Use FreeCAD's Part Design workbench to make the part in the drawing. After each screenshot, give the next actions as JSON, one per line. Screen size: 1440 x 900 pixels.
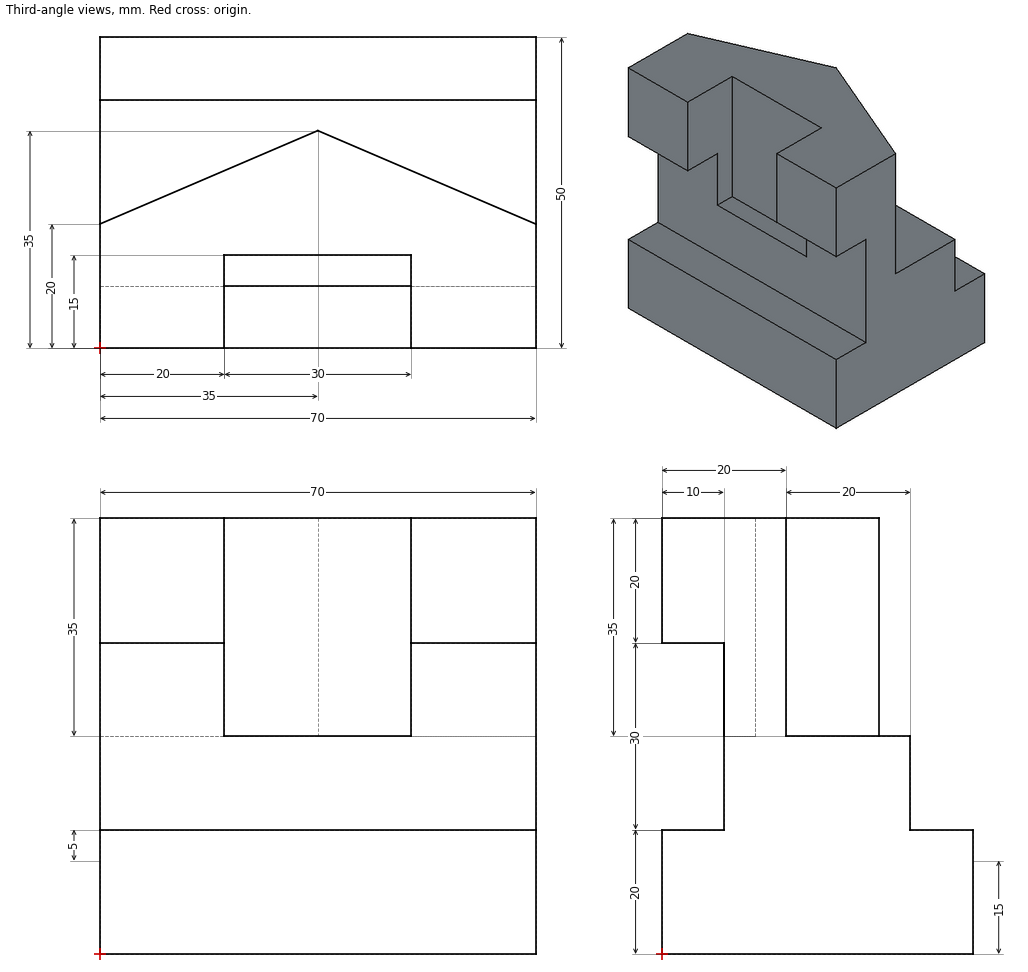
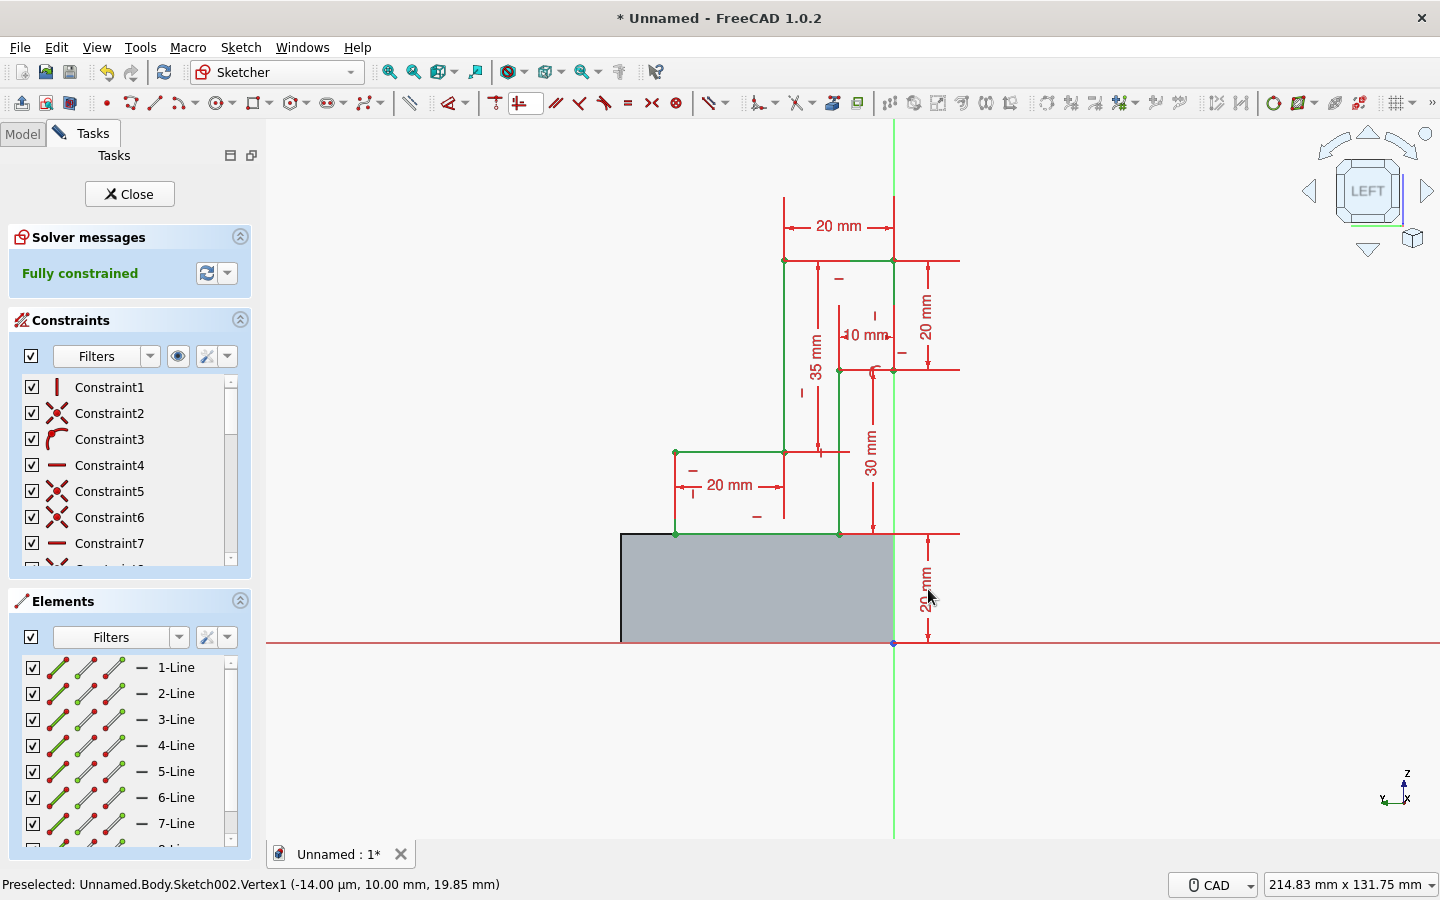
{"action": "left_click", "coordinate": [130, 194]}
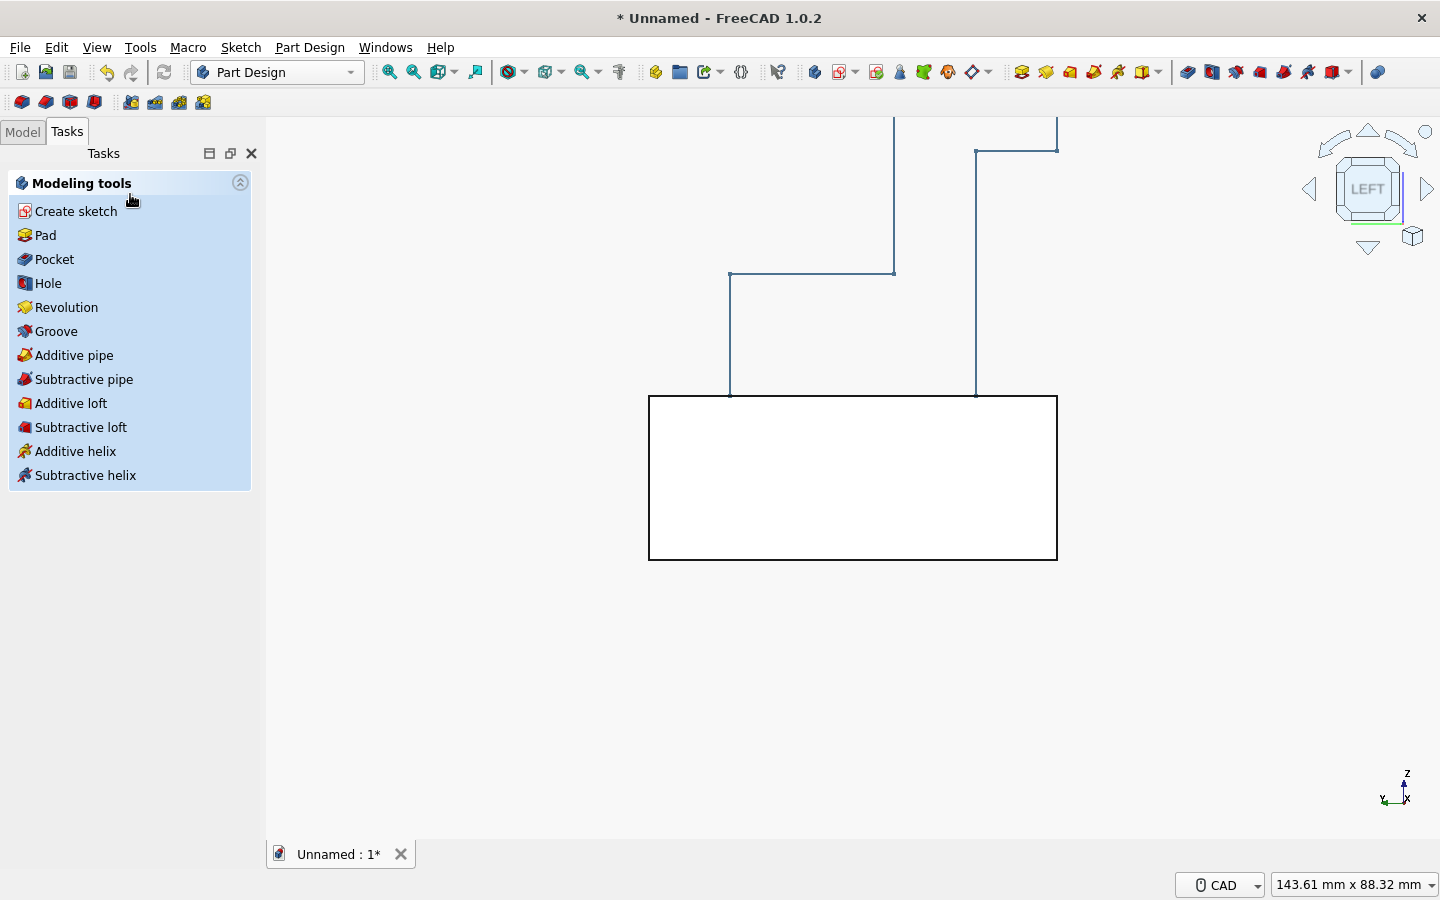
{"action": "left_click", "coordinate": [1022, 72]}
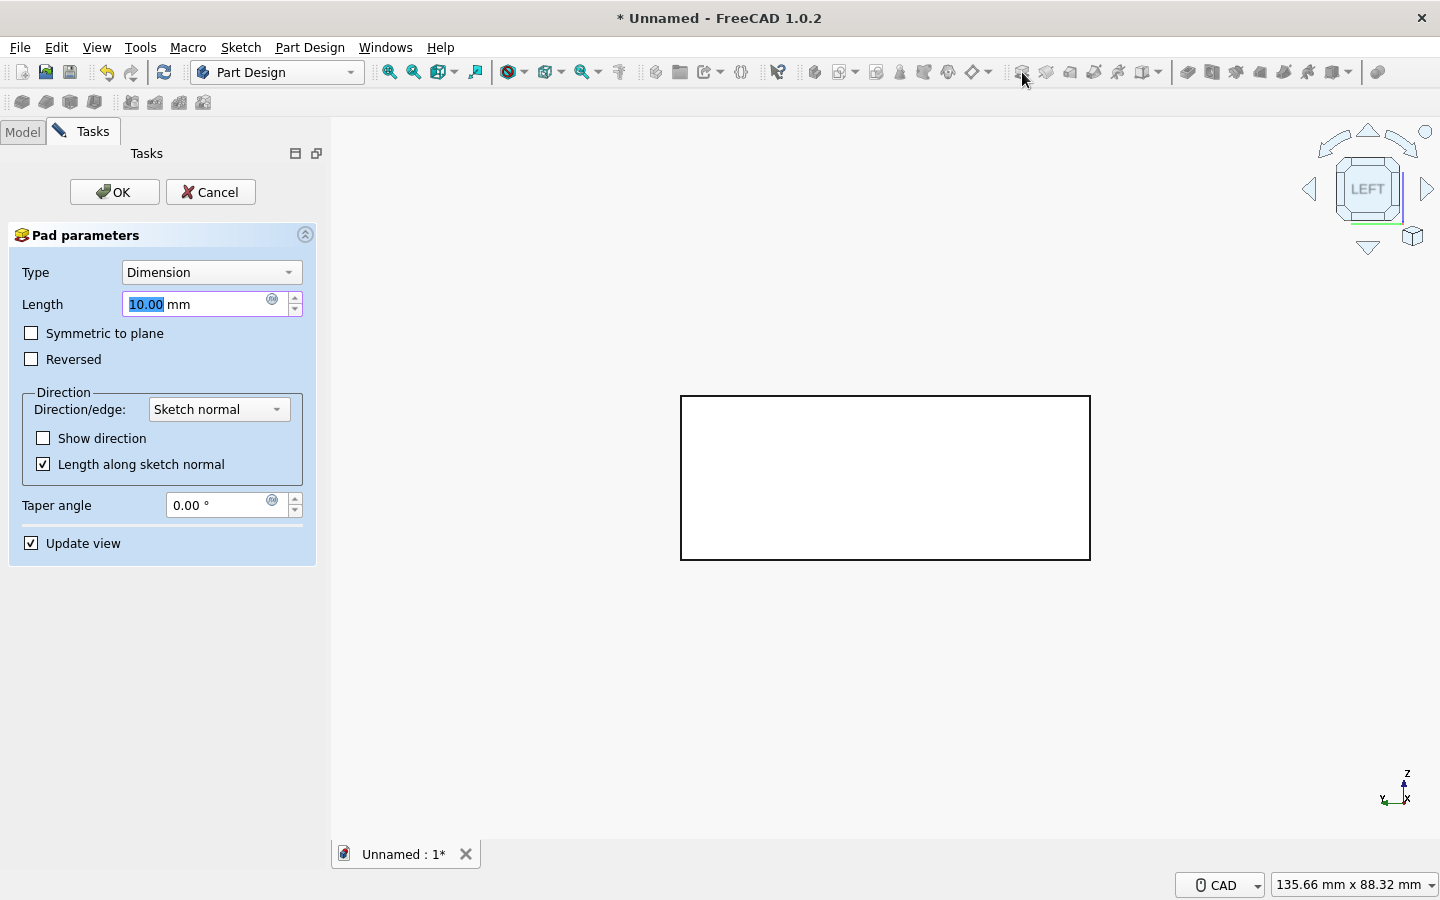
{"action": "type", "text": "70"}
{"action": "key", "text": "Tab"}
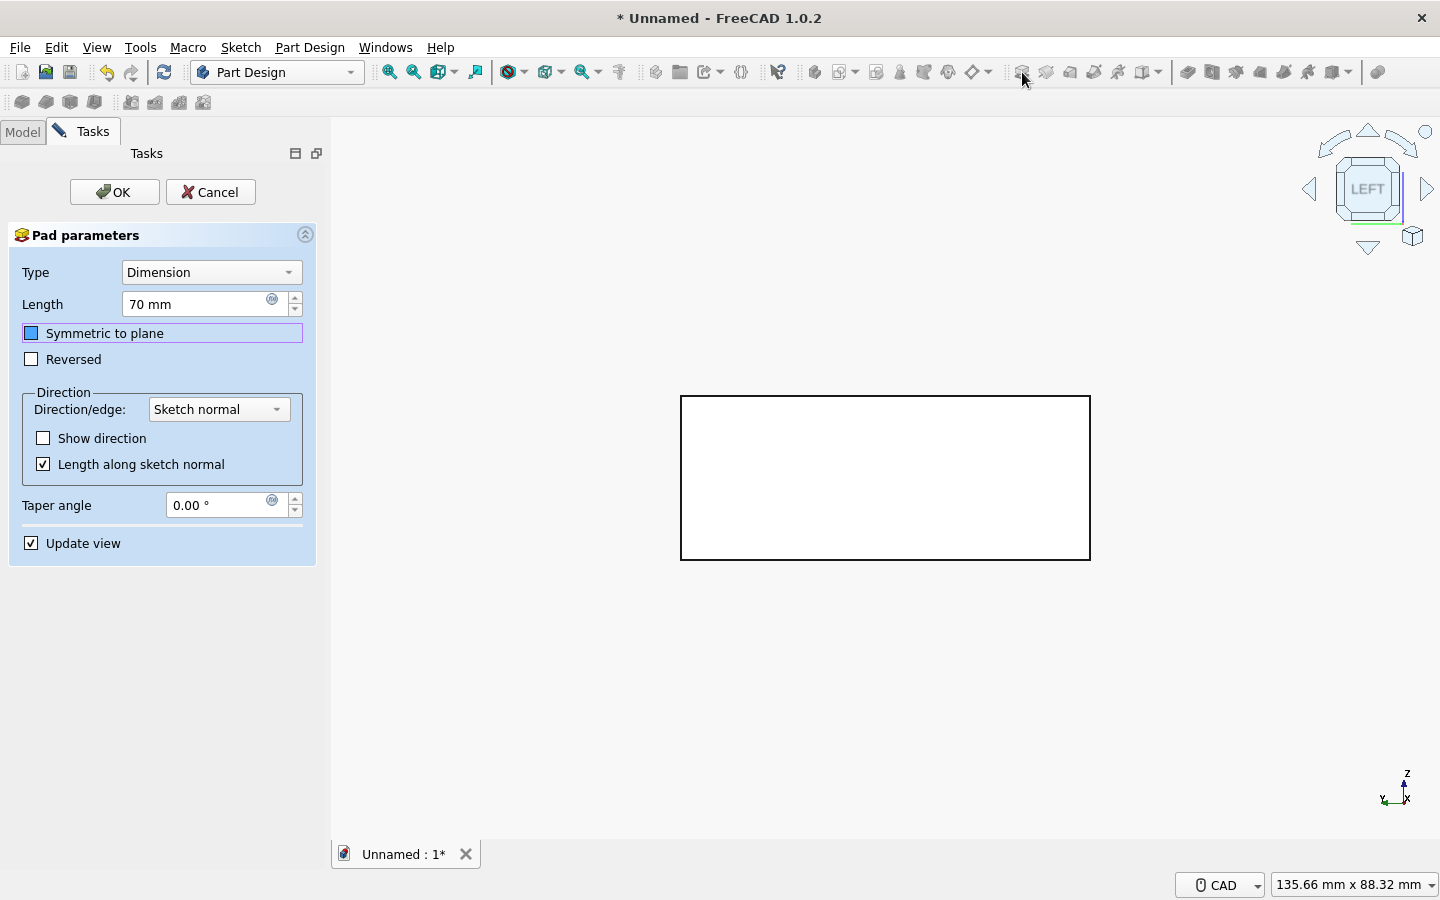
{"action": "left_click", "coordinate": [30, 359]}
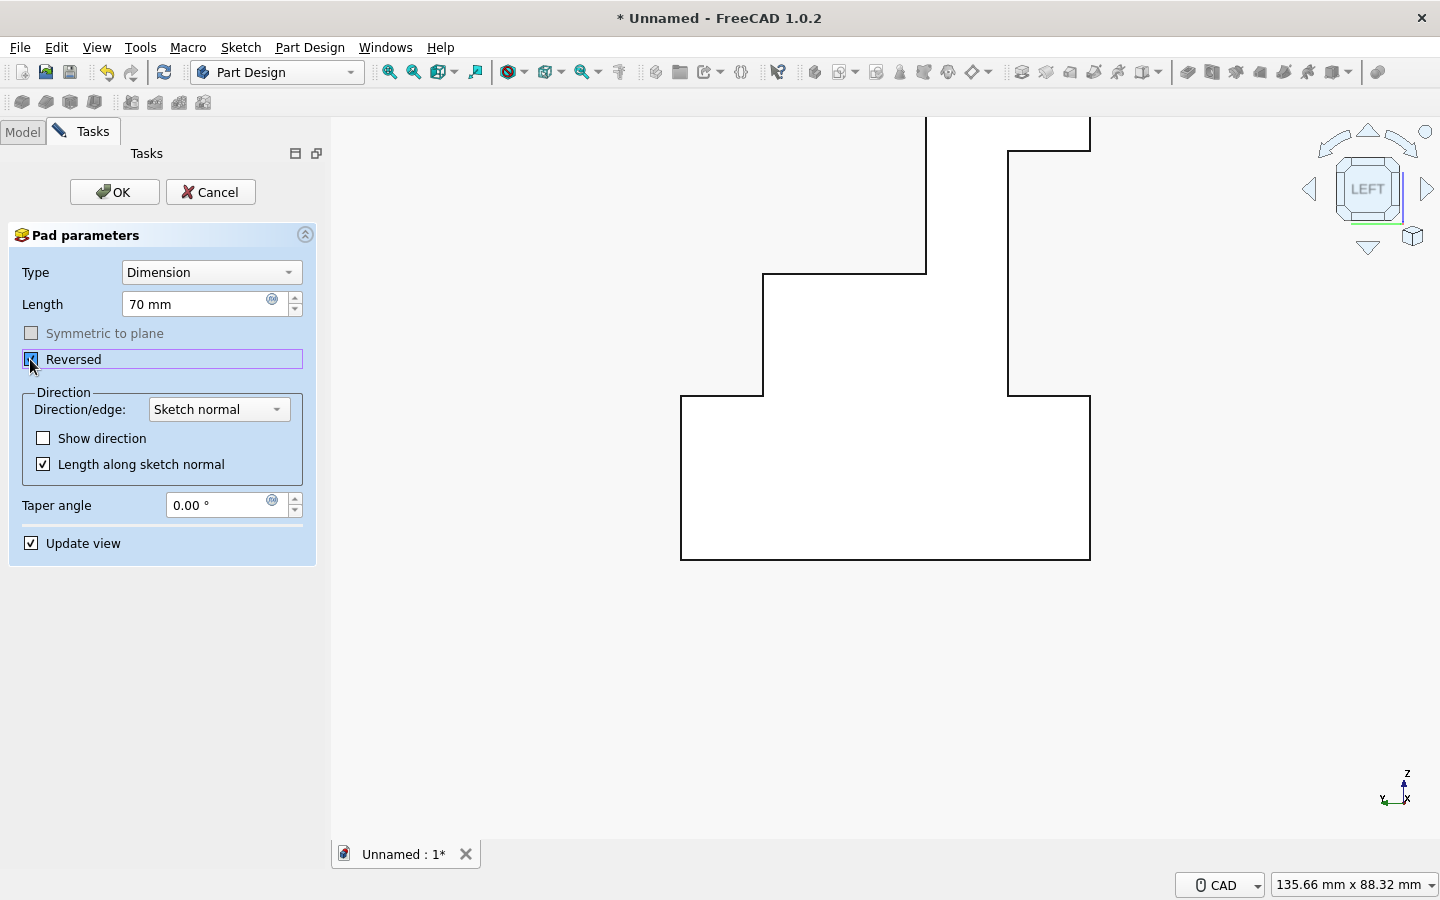
{"action": "left_click", "coordinate": [115, 192]}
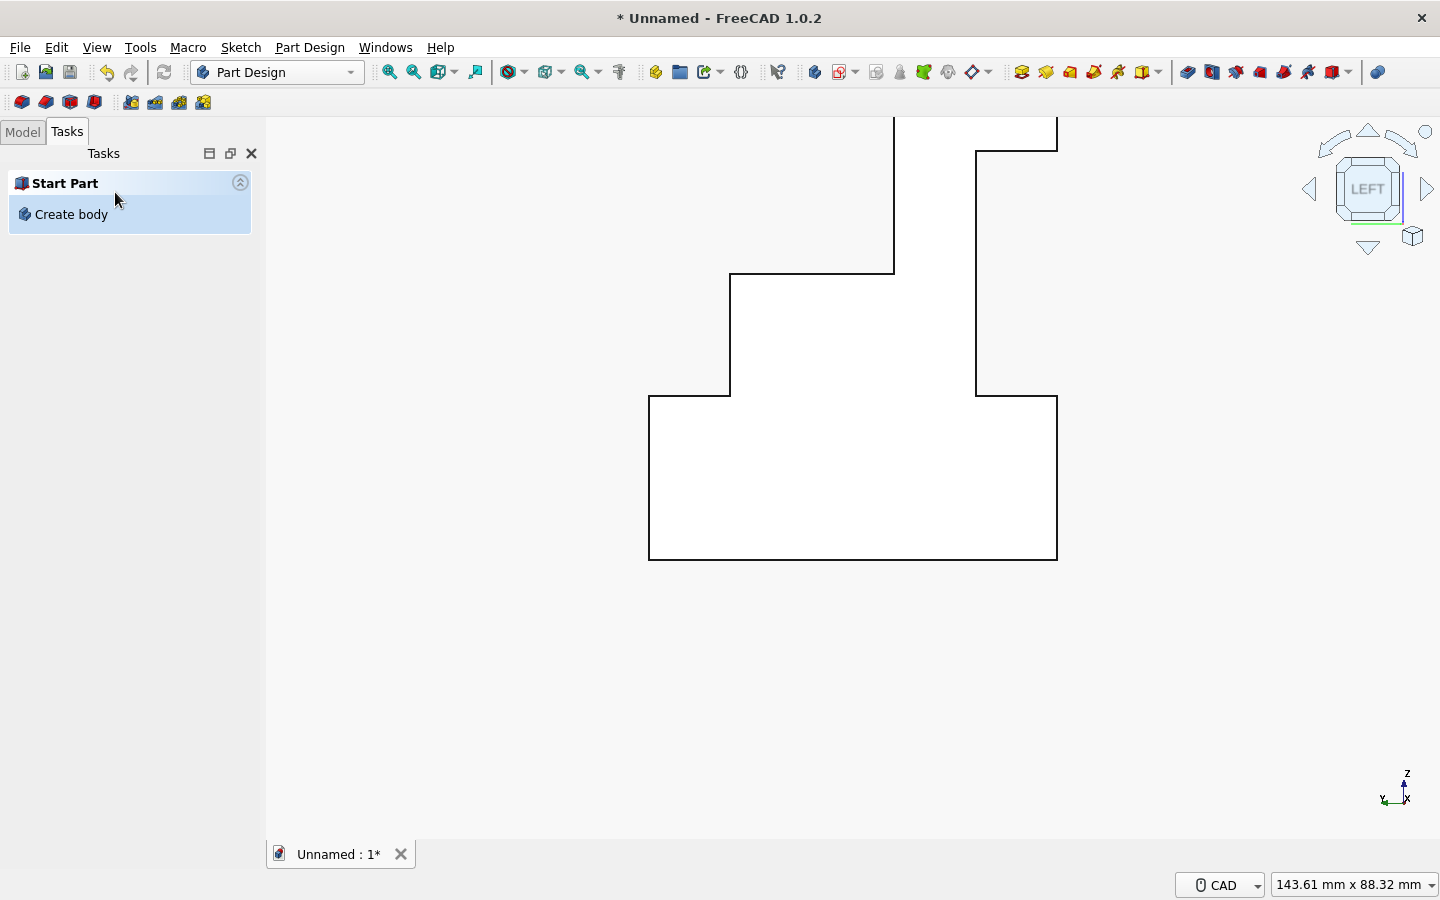
{"action": "left_click", "coordinate": [390, 72]}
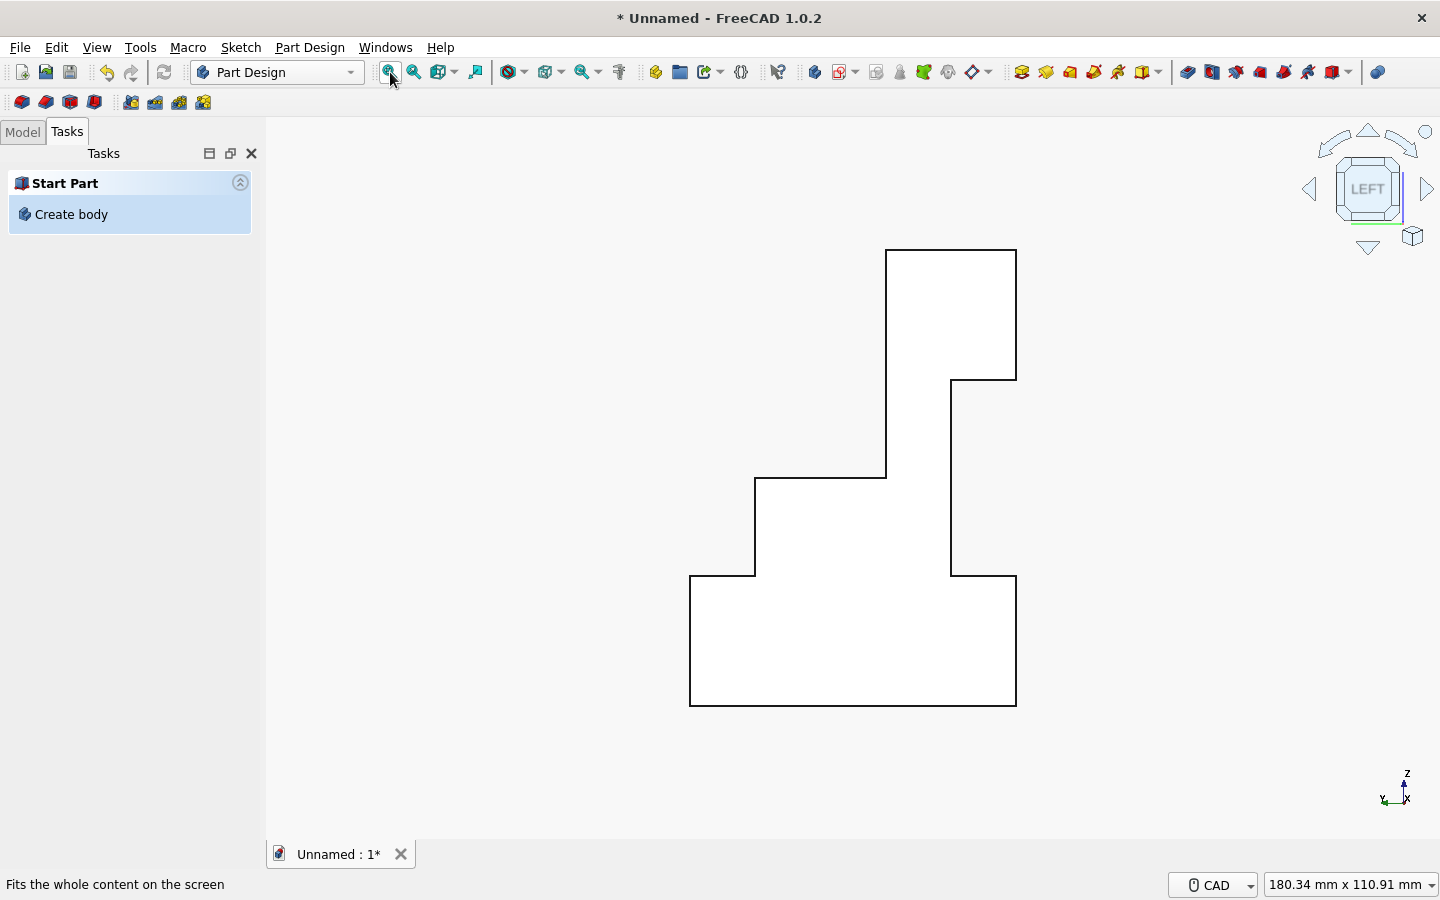
{"action": "key", "text": "0"}